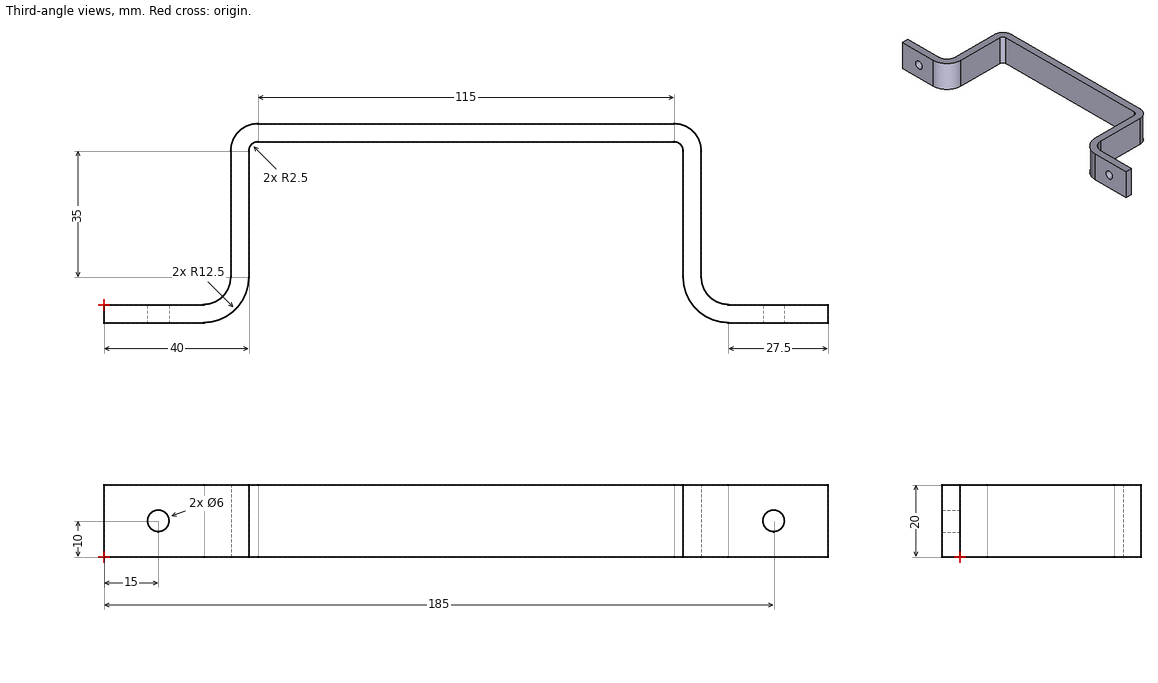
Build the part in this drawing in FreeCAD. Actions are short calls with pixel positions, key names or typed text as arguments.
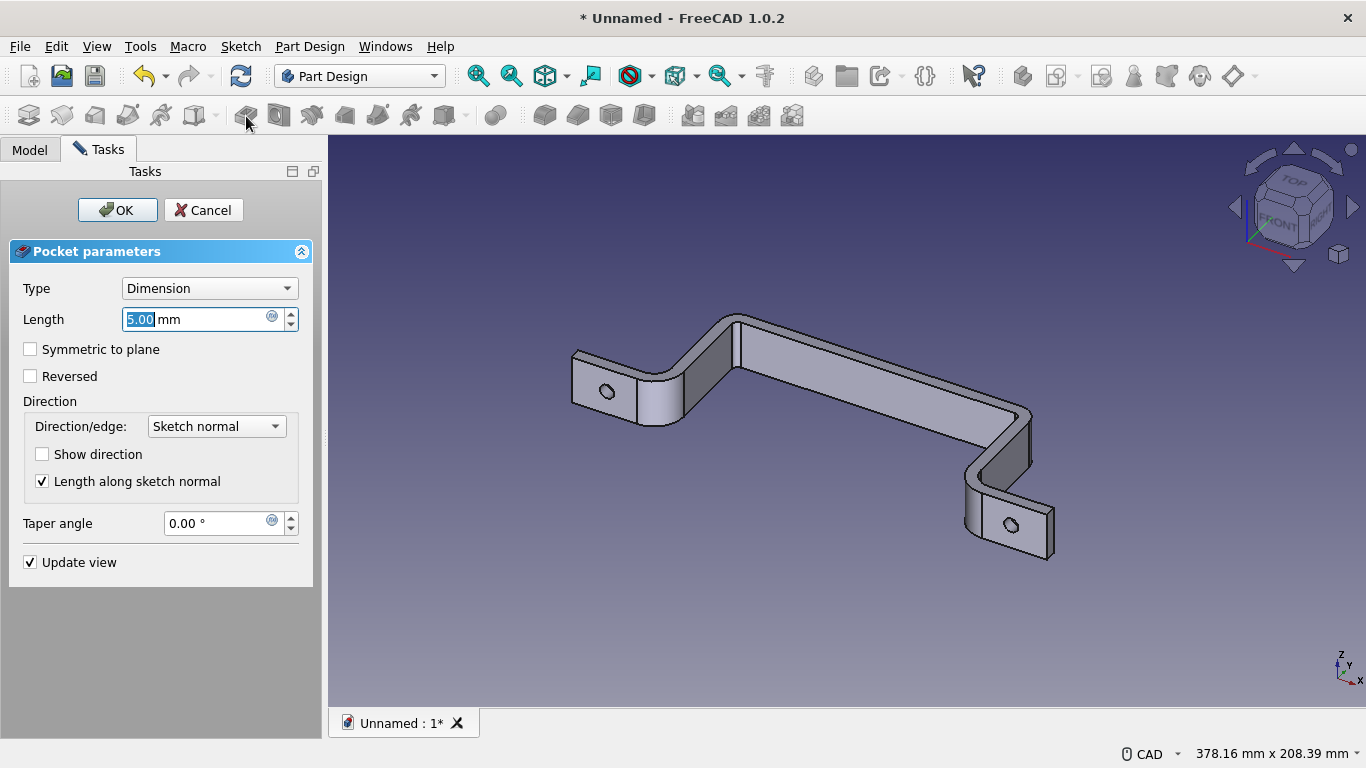
click(210, 288)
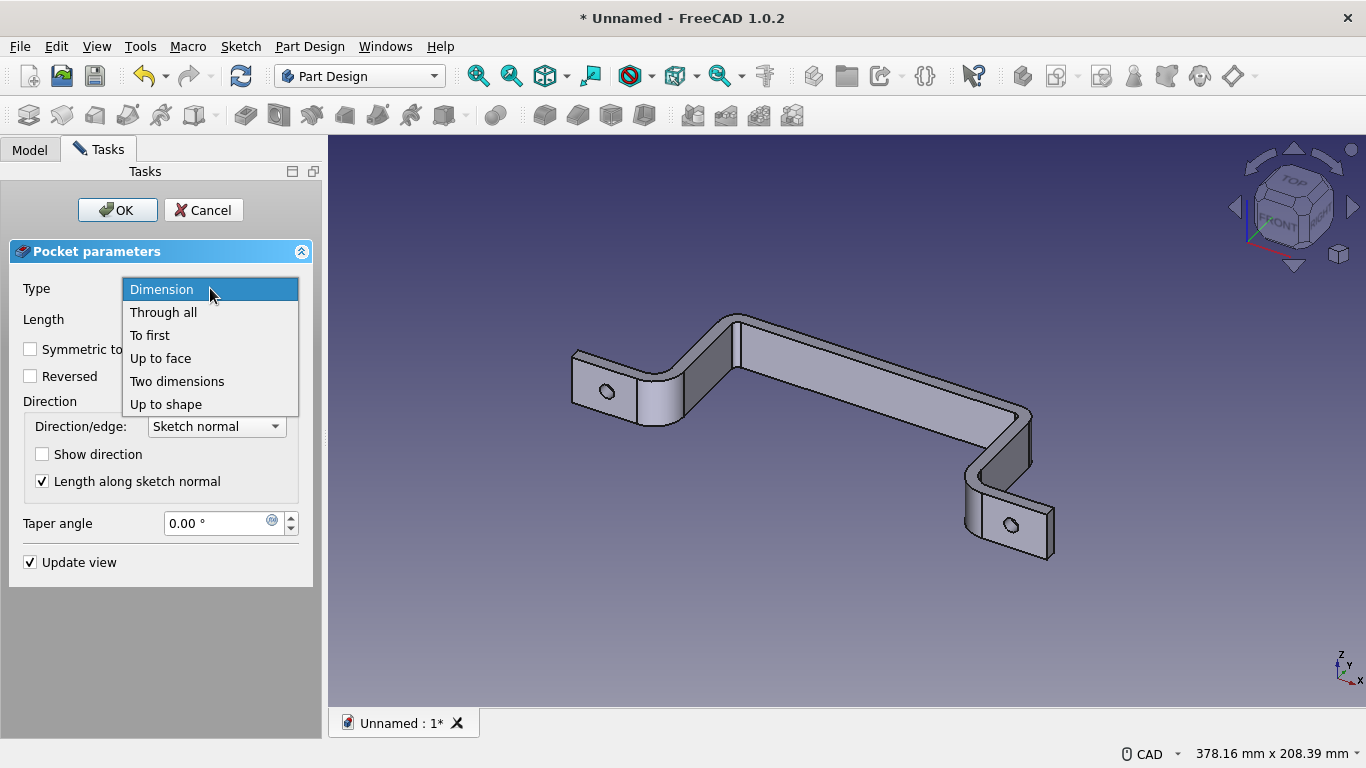
click(208, 312)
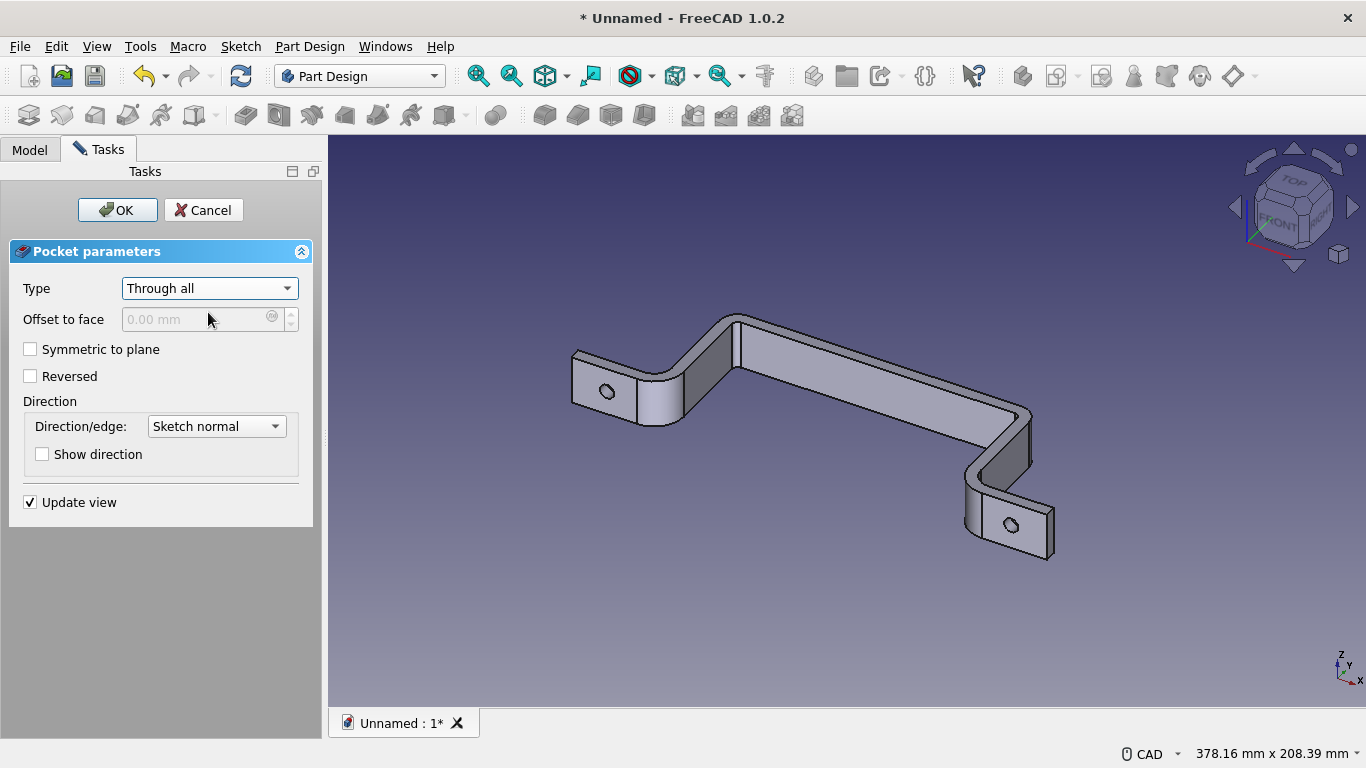
click(118, 210)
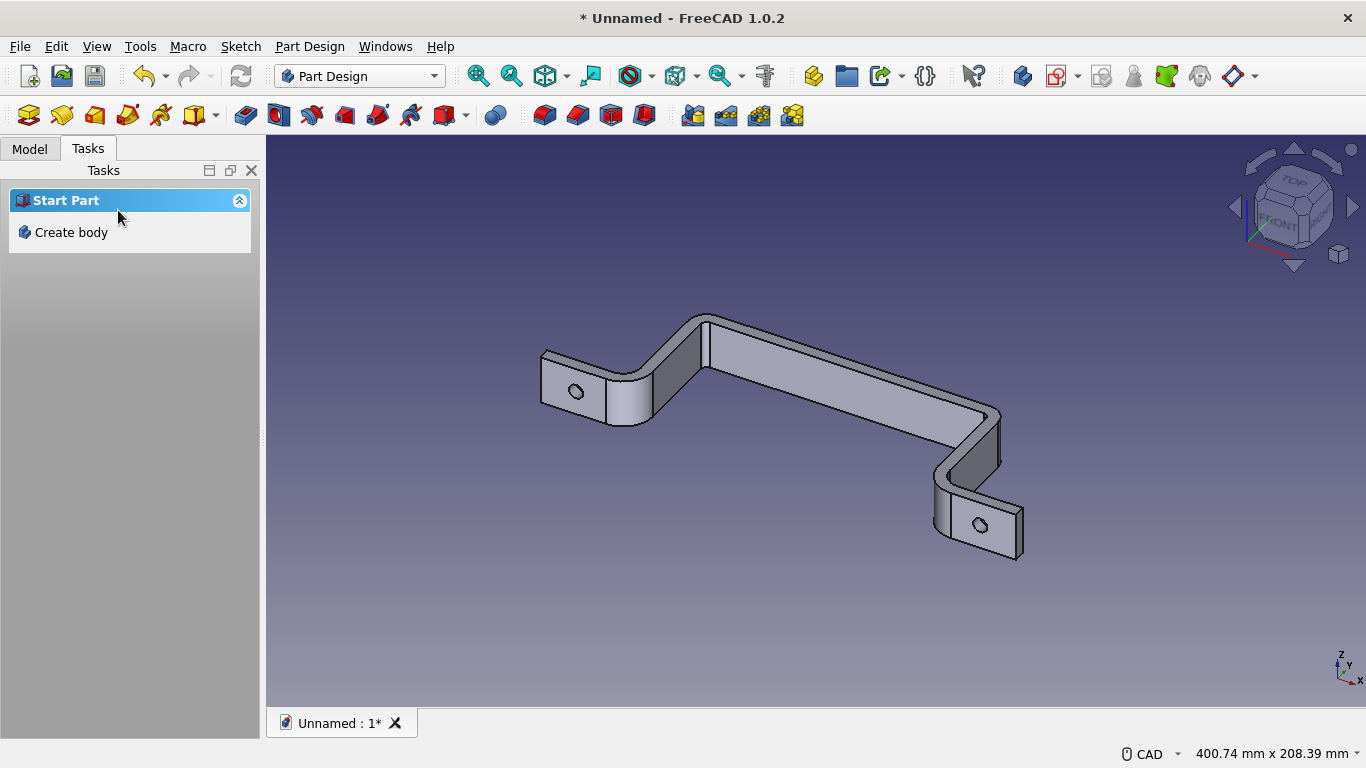
key(0)